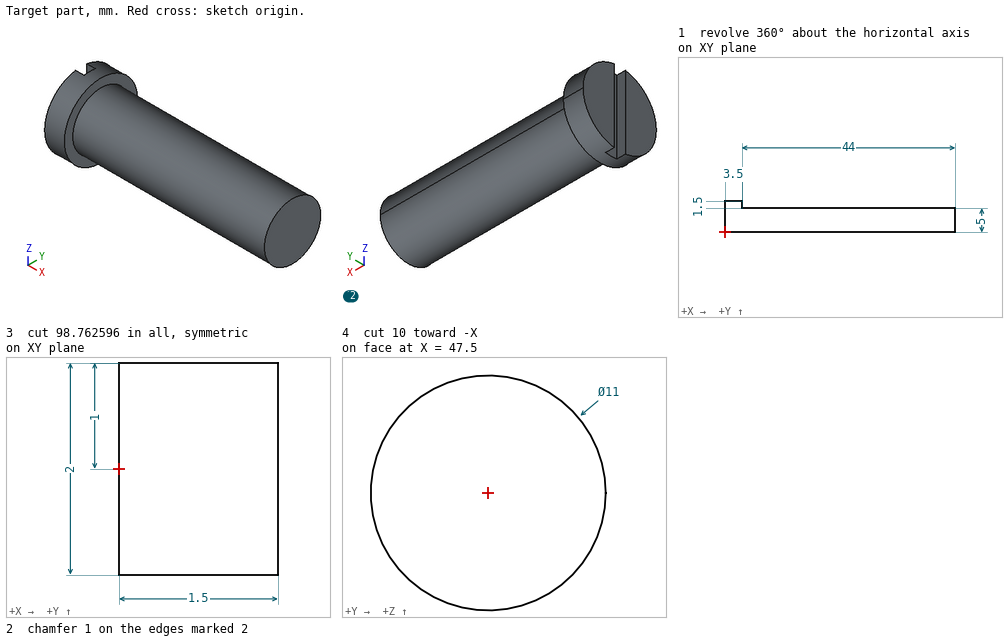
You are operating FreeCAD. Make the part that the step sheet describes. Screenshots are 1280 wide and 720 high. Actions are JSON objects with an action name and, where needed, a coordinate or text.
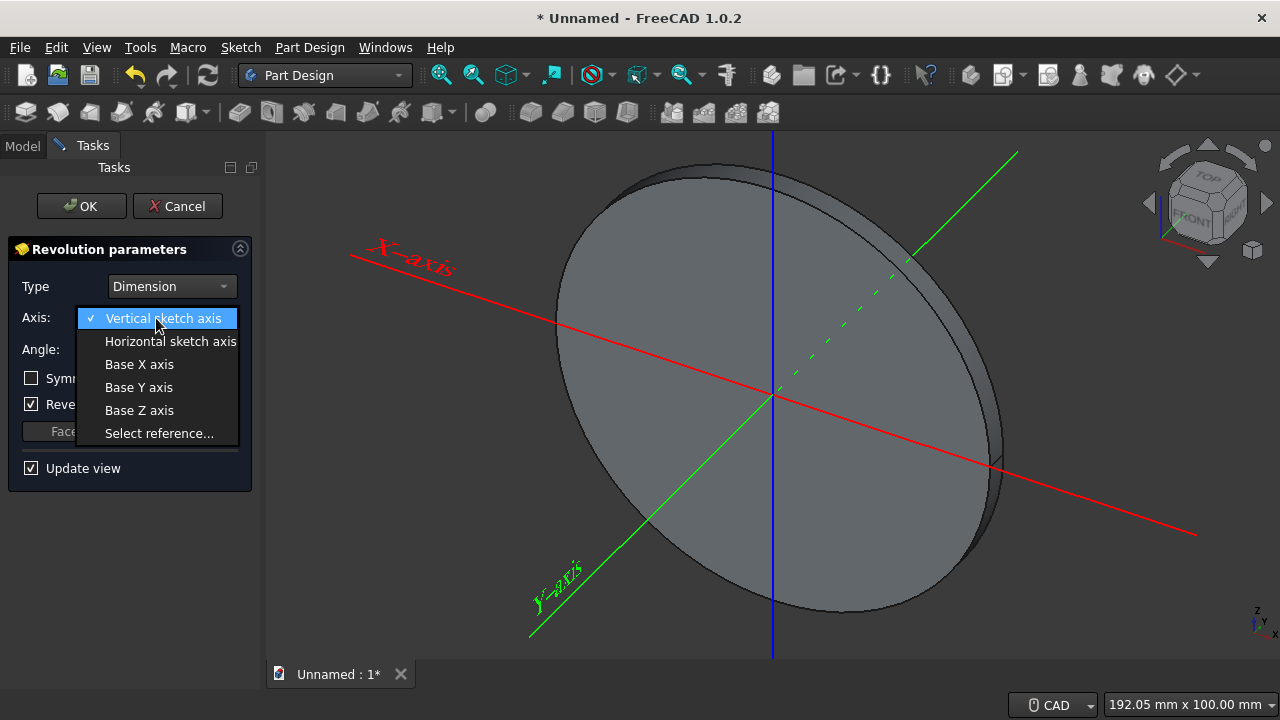
{"action": "left_click", "coordinate": [156, 342]}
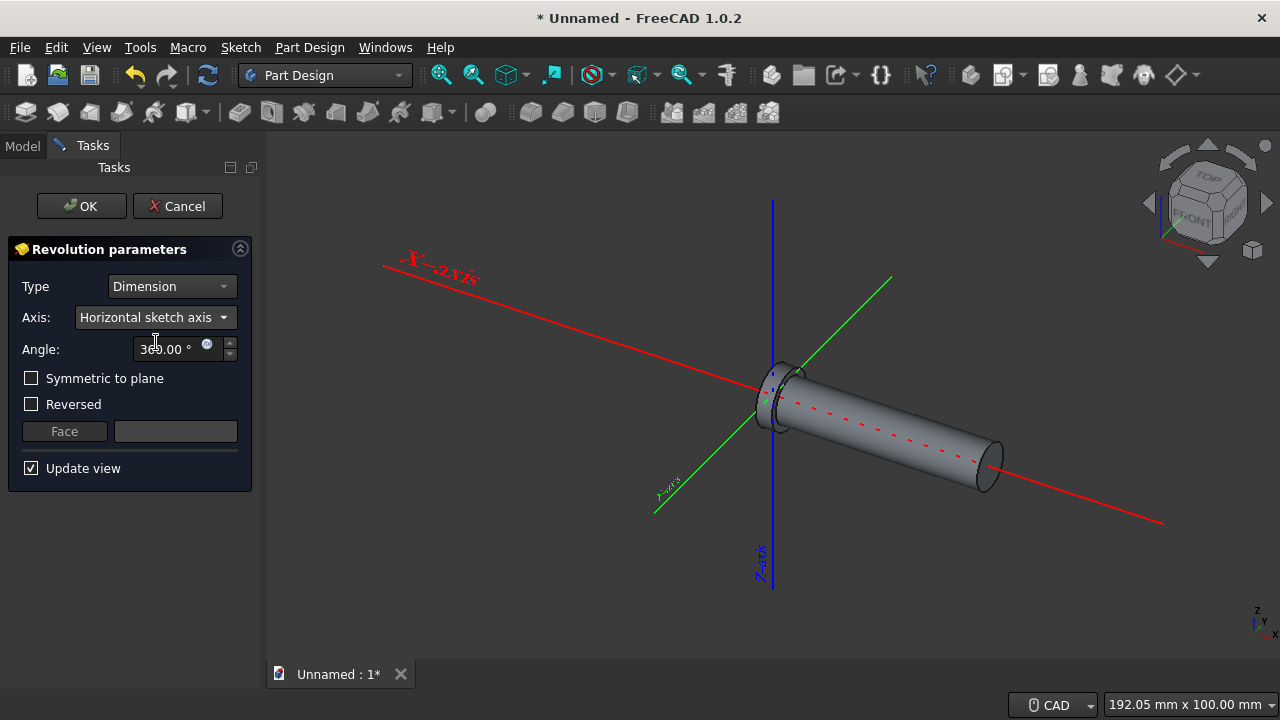
{"action": "left_click", "coordinate": [82, 206]}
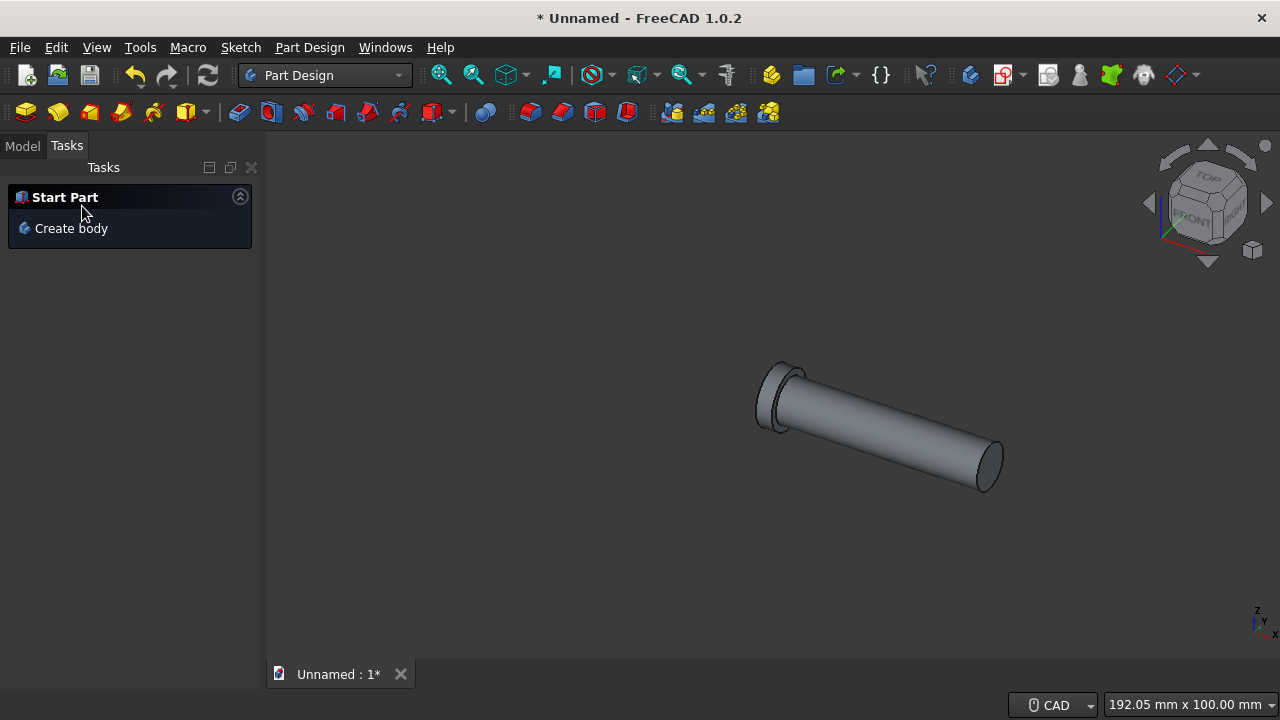
{"action": "left_click", "coordinate": [442, 76]}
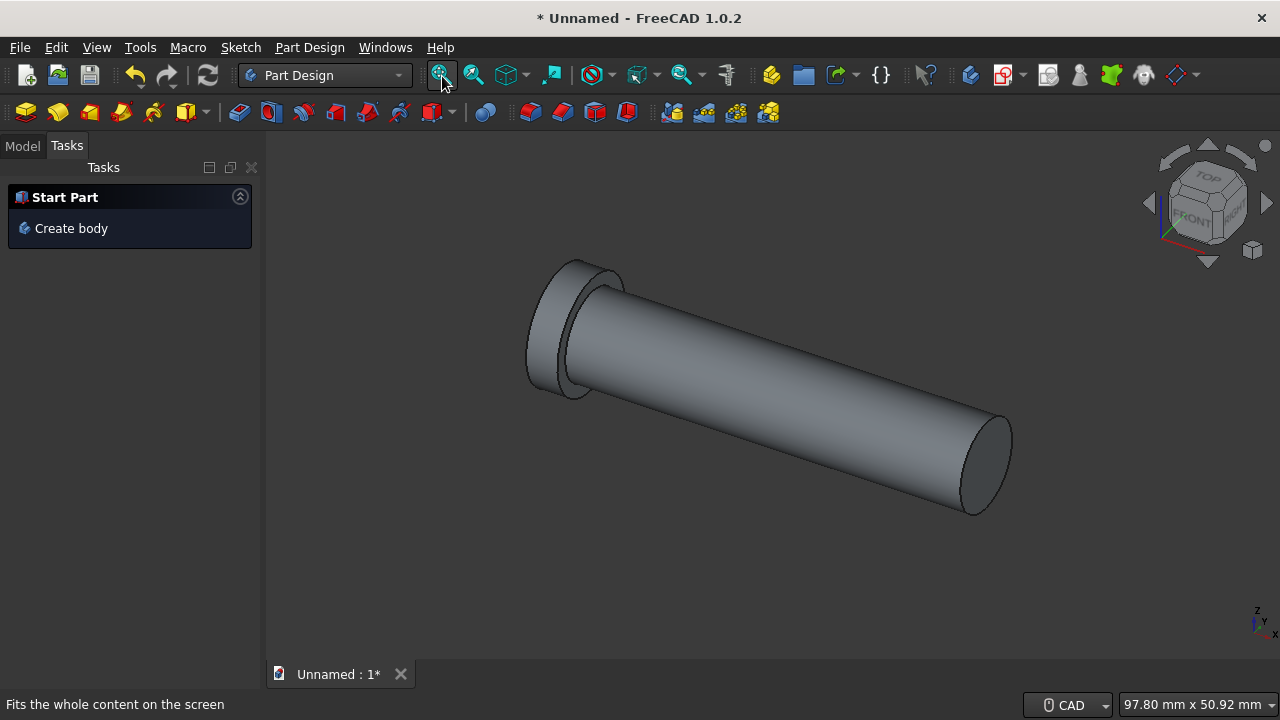
{"action": "left_click", "coordinate": [960, 490]}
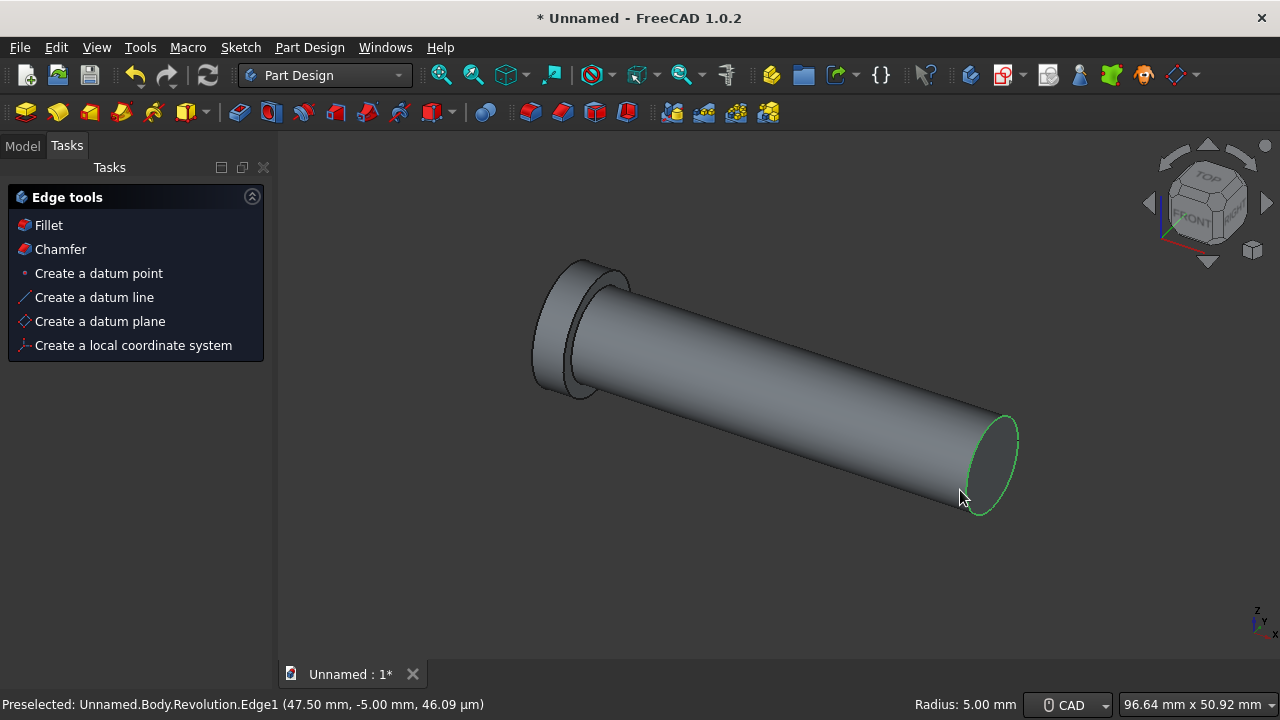
{"action": "left_click", "coordinate": [564, 112]}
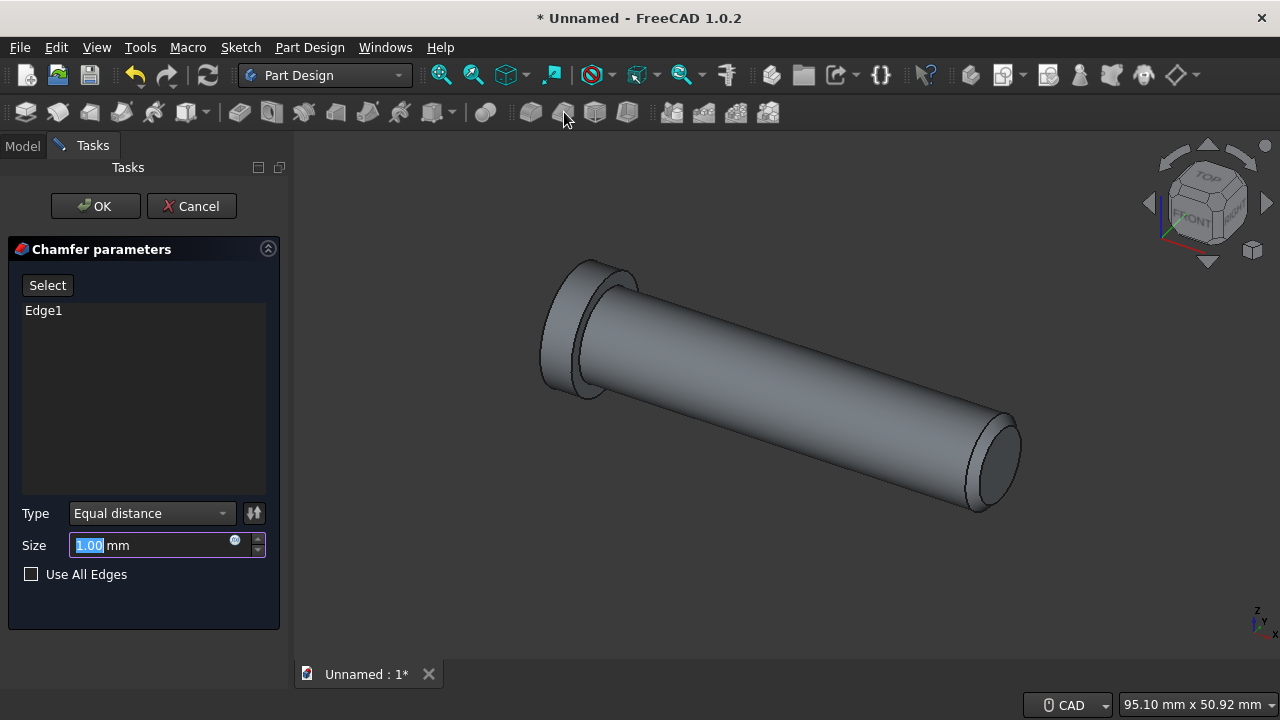
{"action": "type", "text": "1"}
{"action": "key", "text": "Tab"}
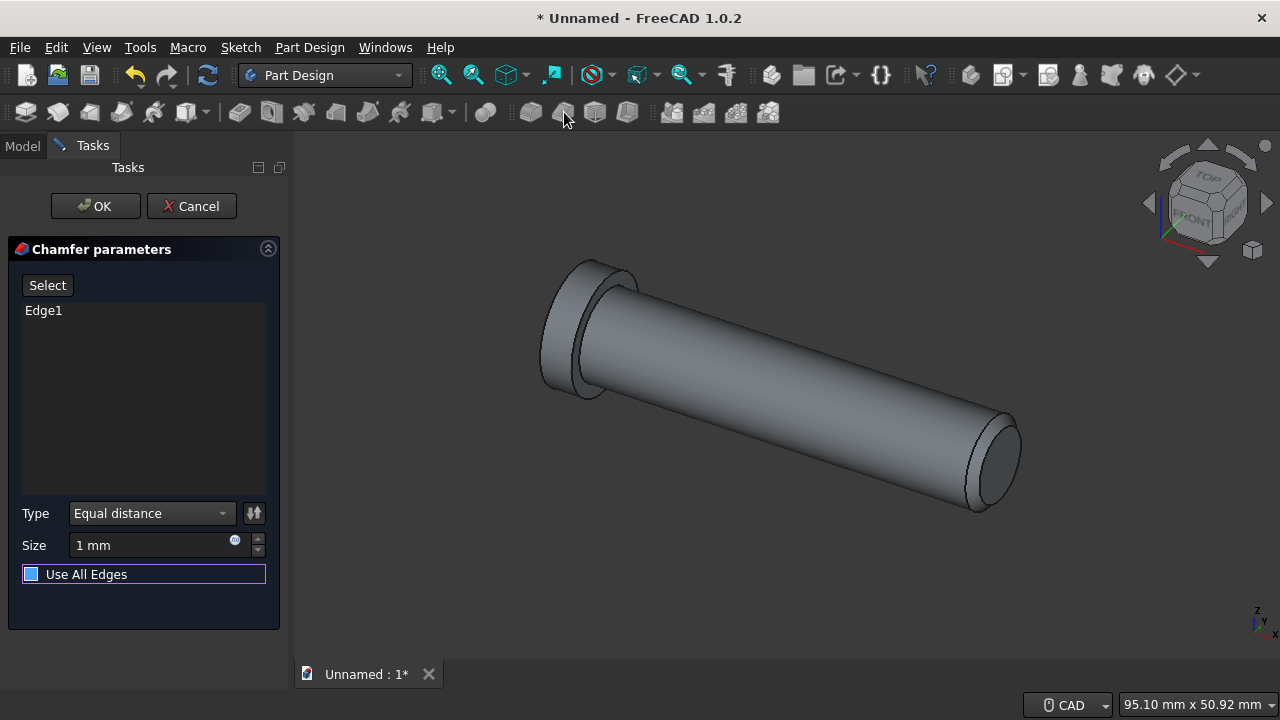
{"action": "left_click", "coordinate": [96, 206]}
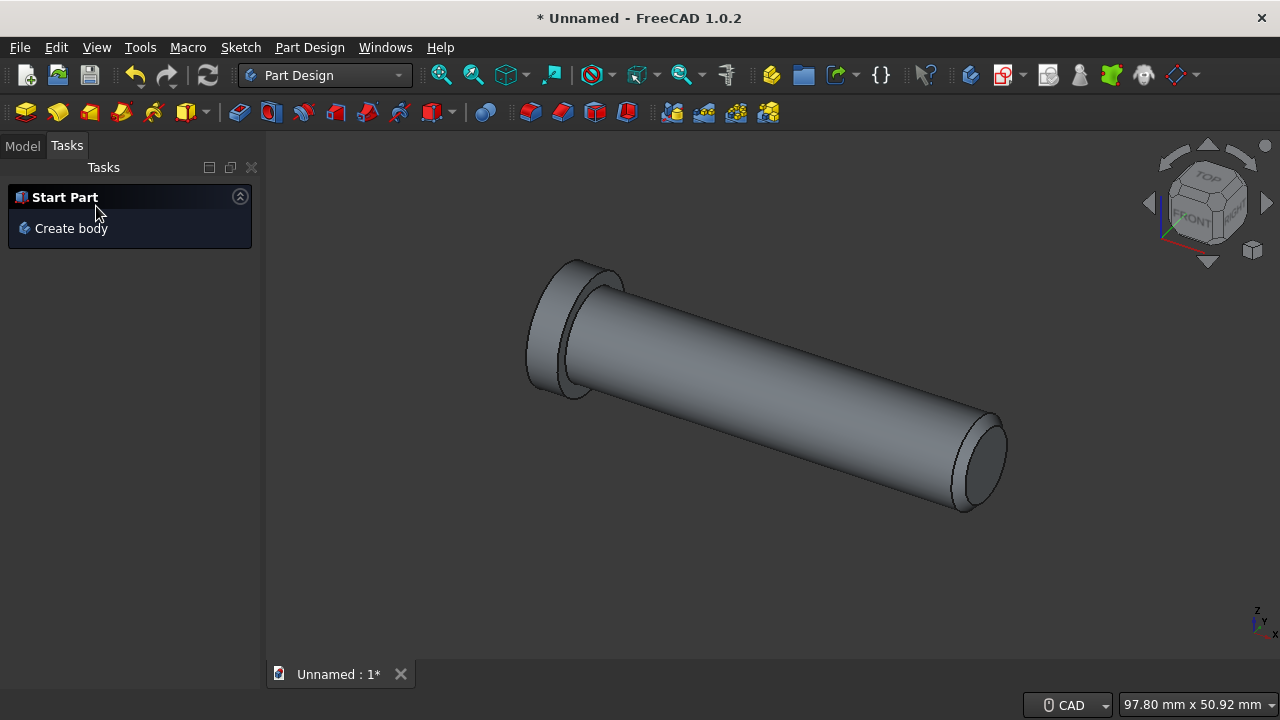
{"action": "left_click", "coordinate": [1004, 76]}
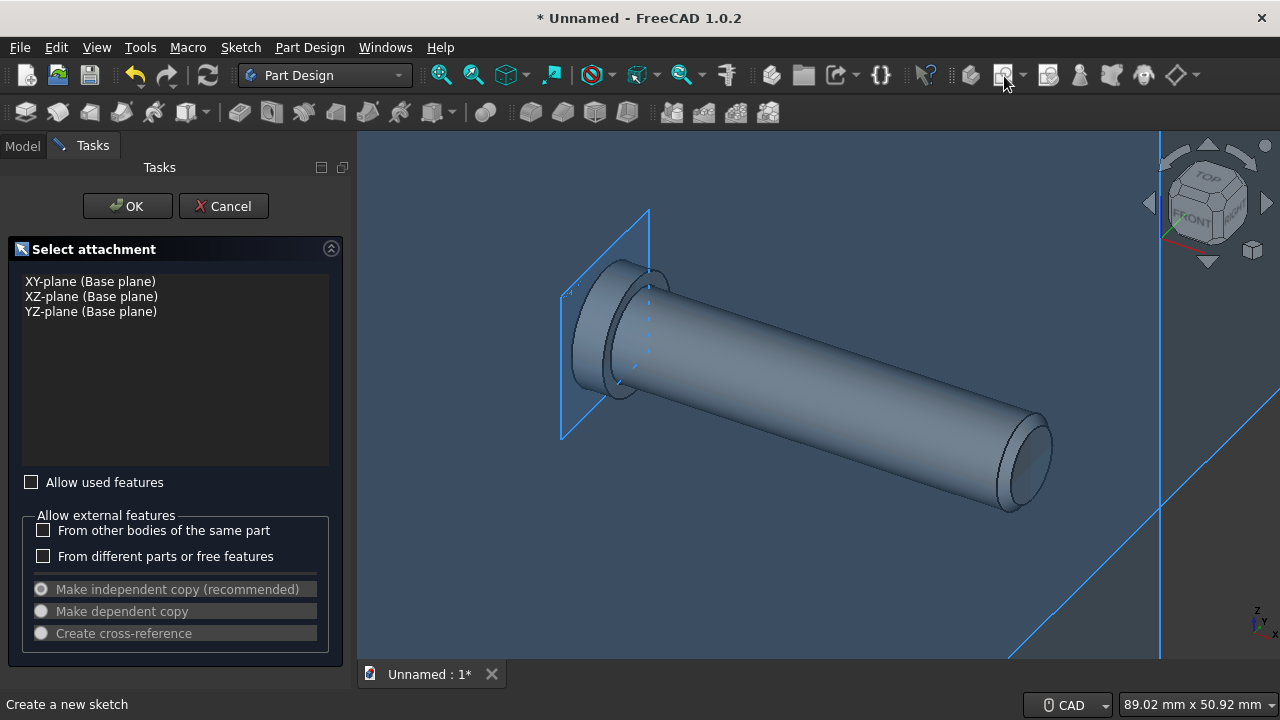
{"action": "left_click", "coordinate": [82, 282]}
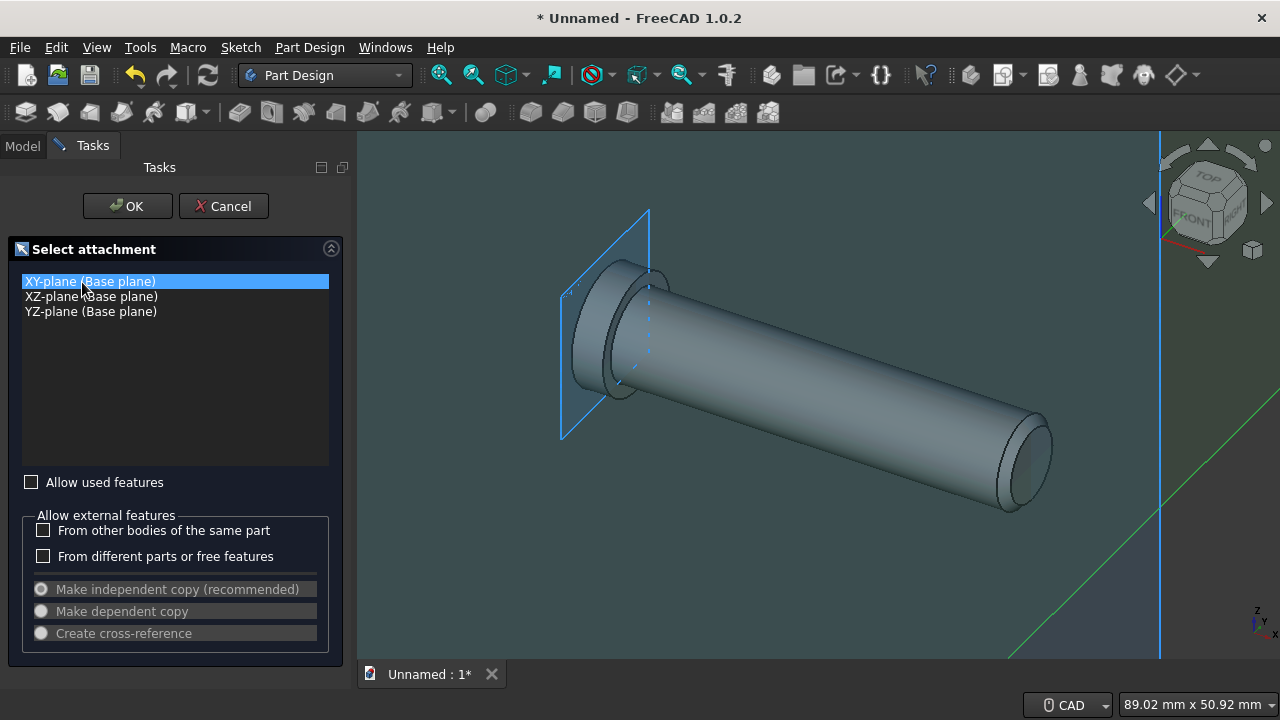
{"action": "left_click", "coordinate": [128, 206]}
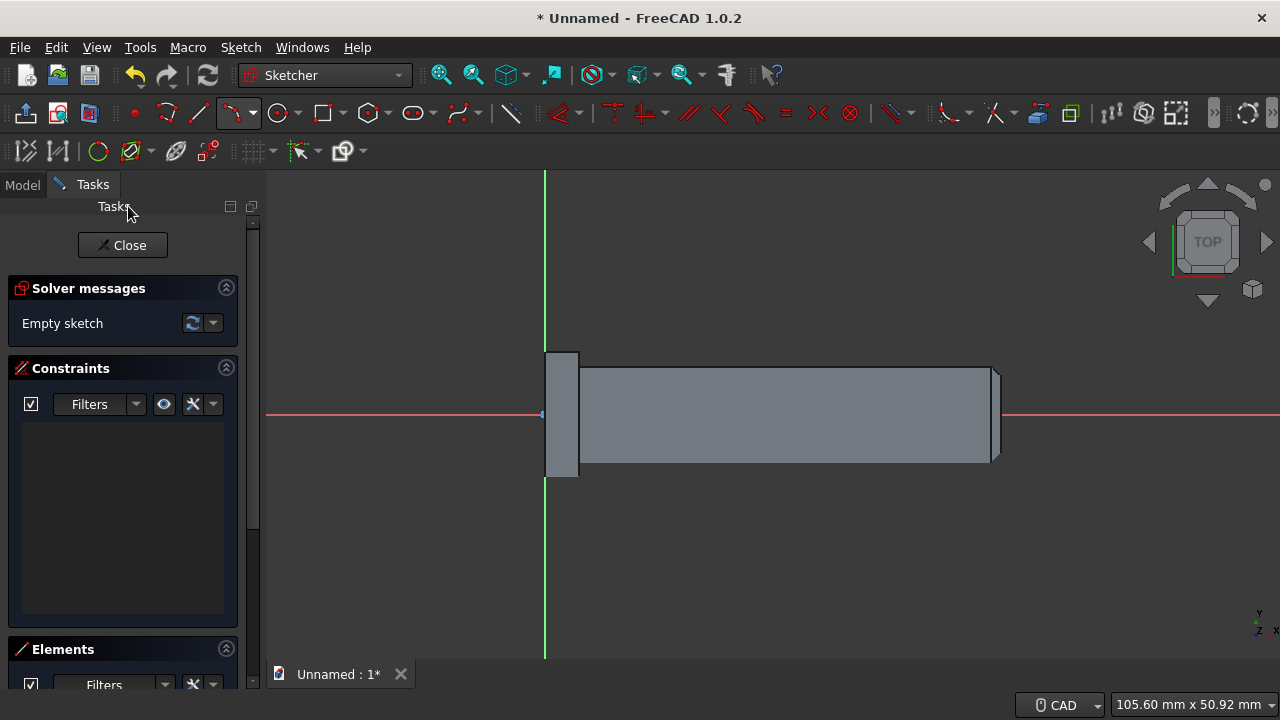
{"action": "key", "text": "q s"}